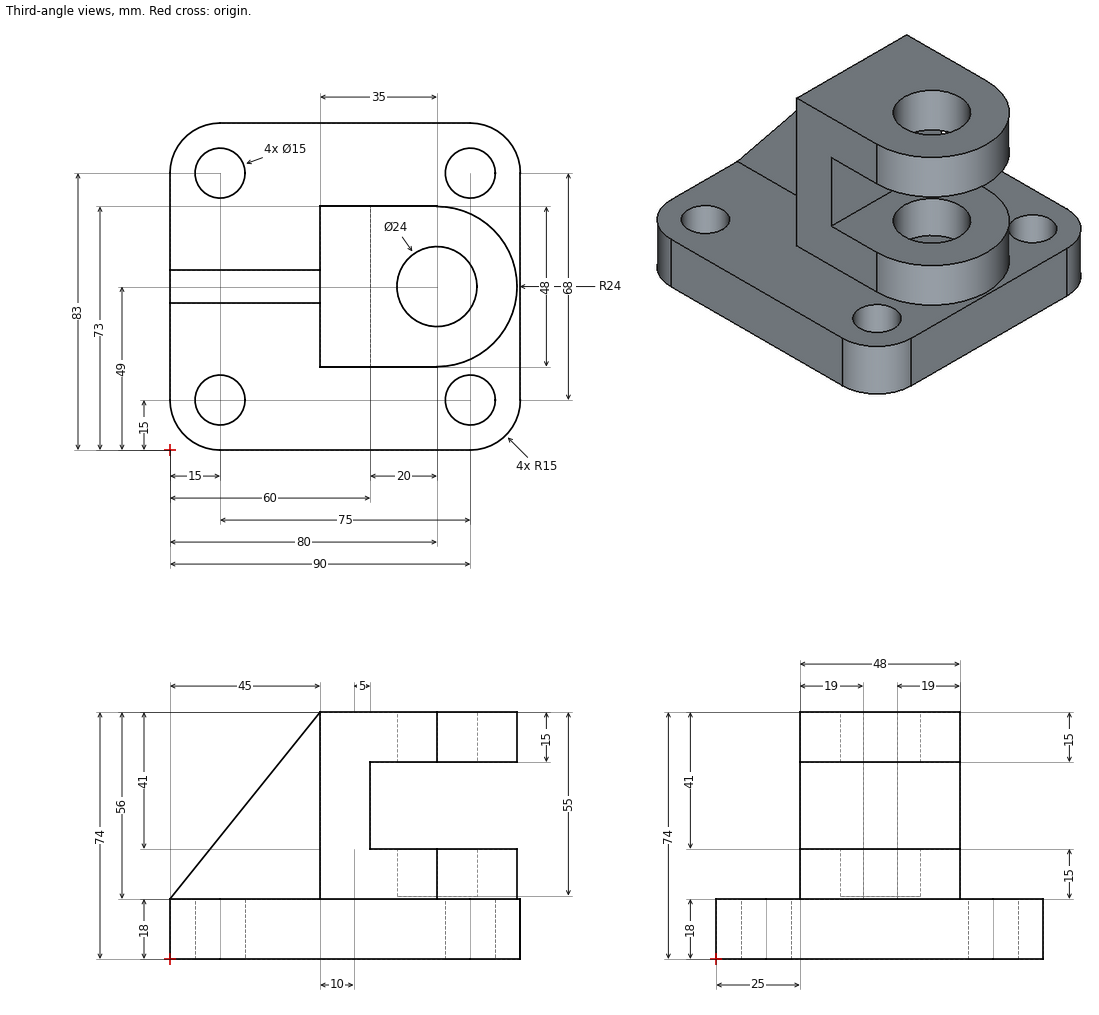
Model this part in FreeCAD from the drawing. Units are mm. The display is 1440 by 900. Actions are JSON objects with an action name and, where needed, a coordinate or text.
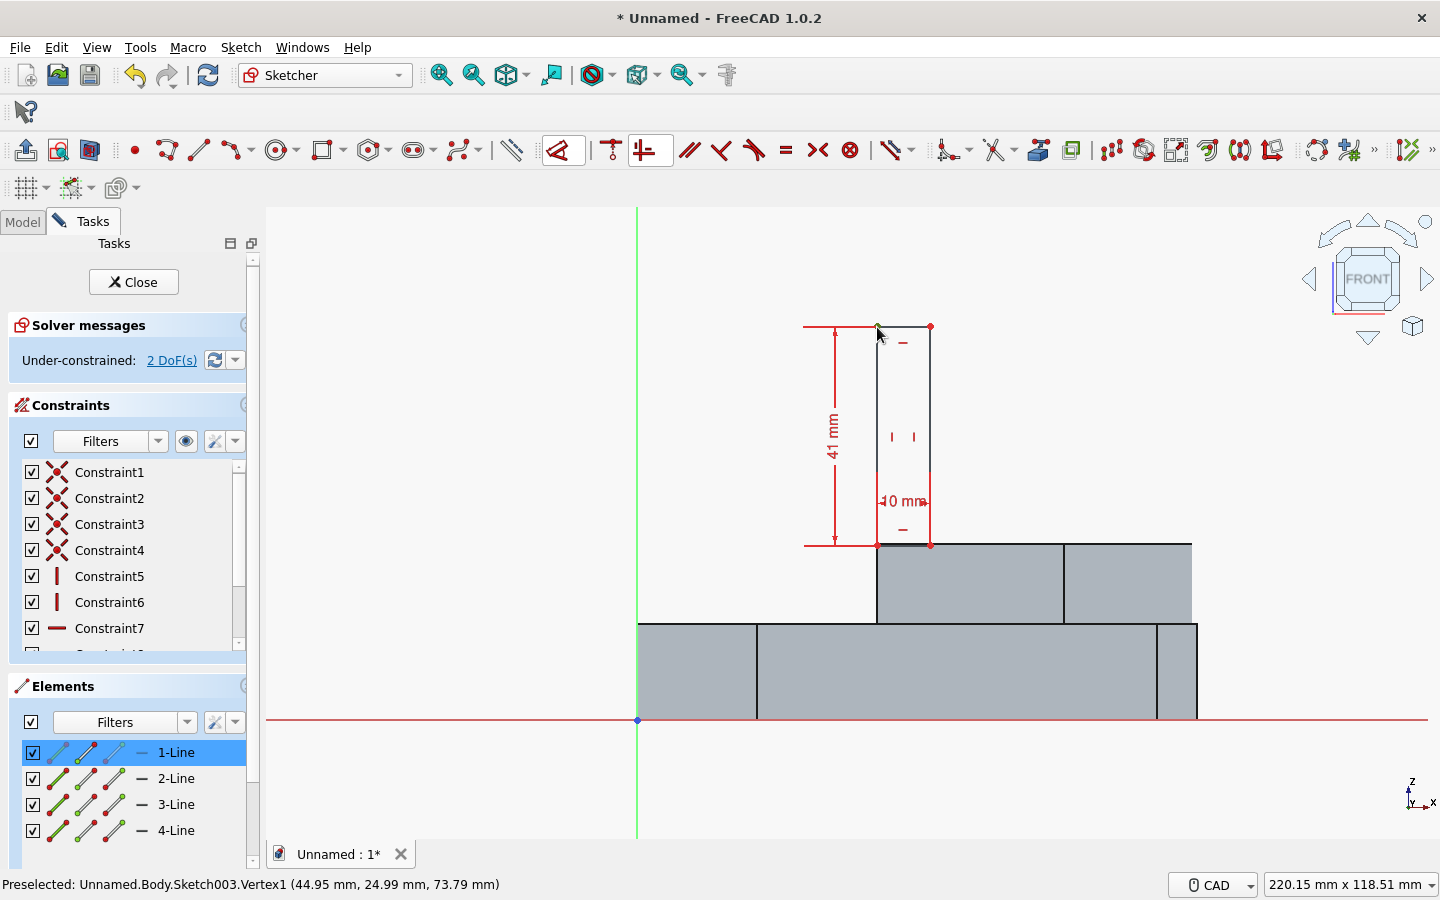
{"action": "left_click", "coordinate": [580, 150]}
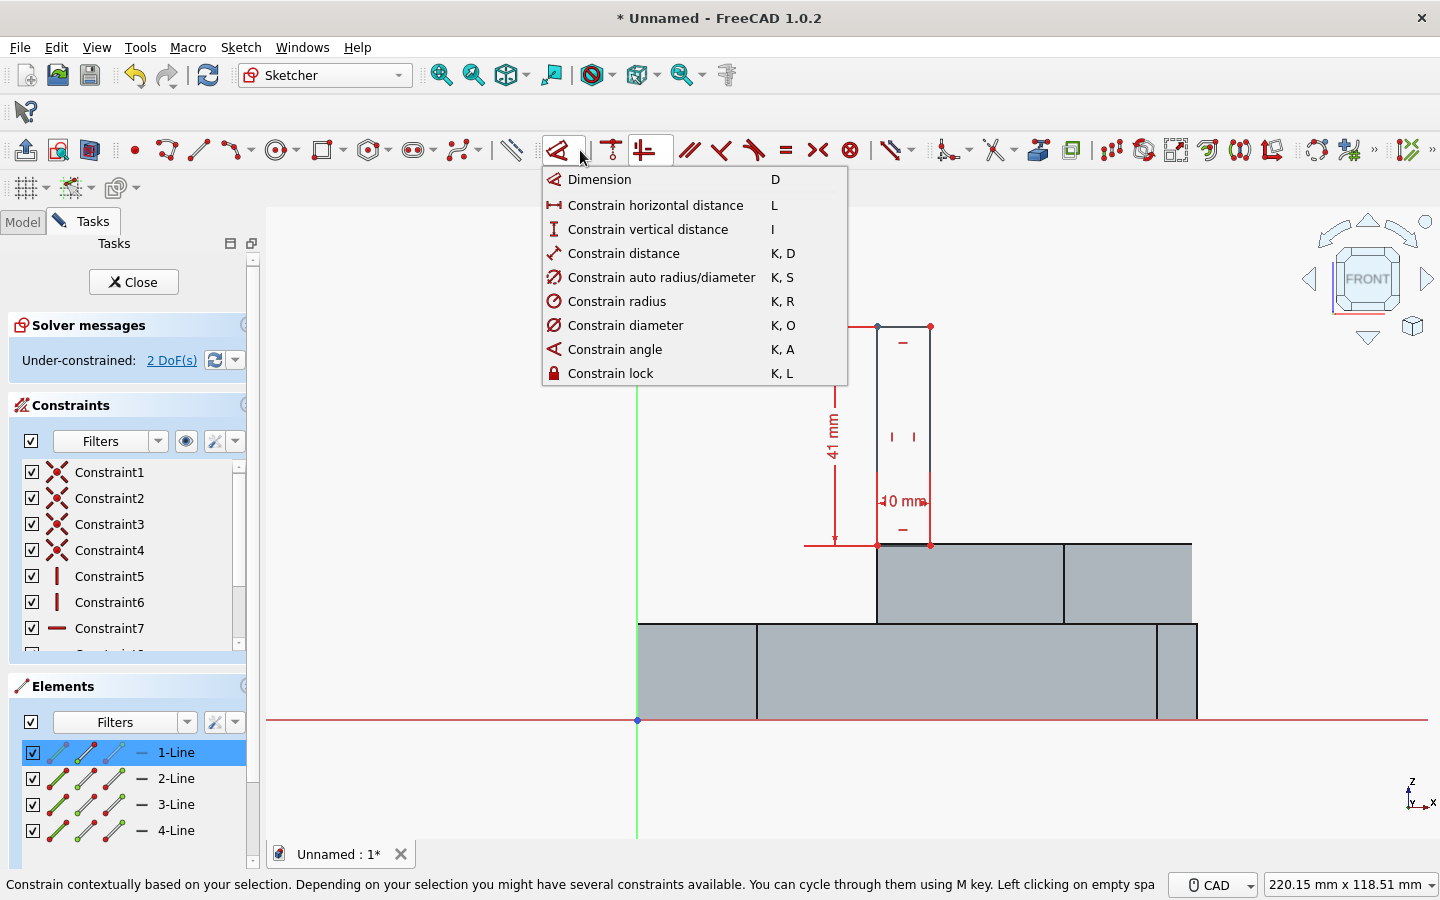
{"action": "left_click", "coordinate": [695, 205]}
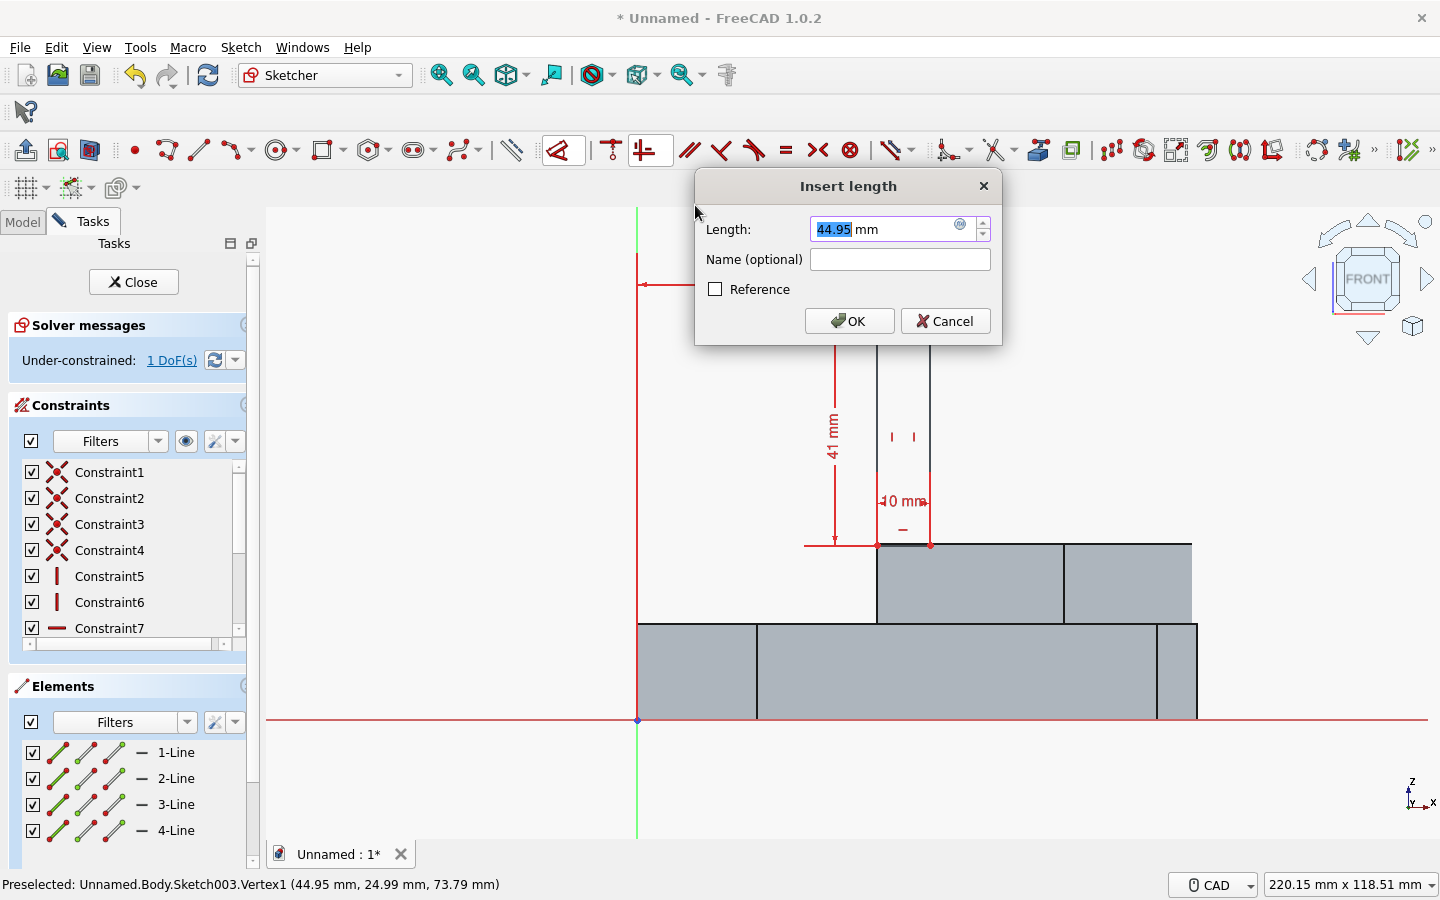
{"action": "type", "text": "45"}
{"action": "key", "text": "Return"}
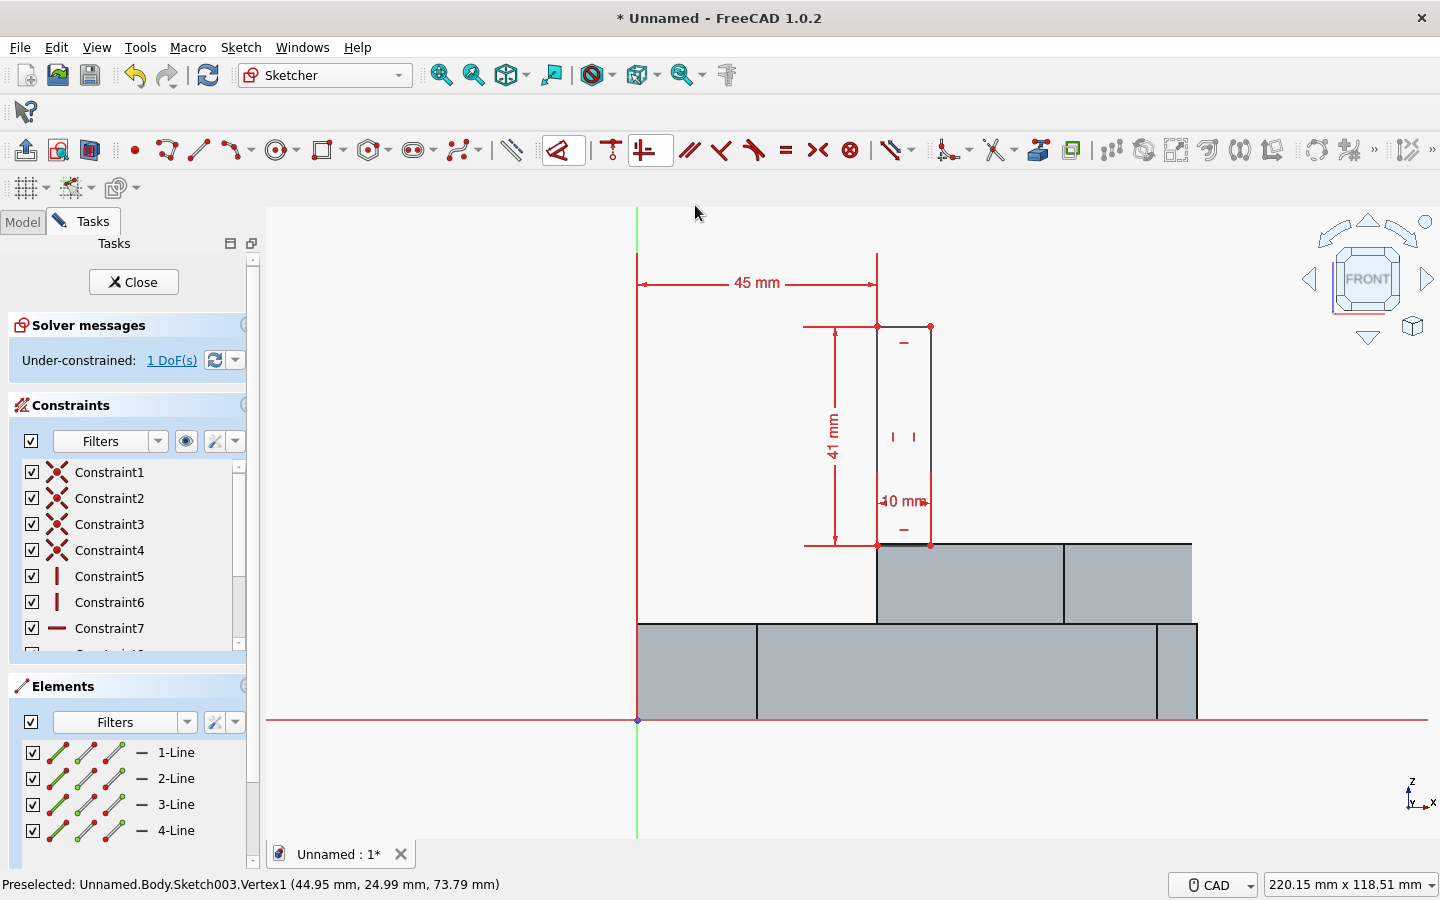
{"action": "left_click", "coordinate": [877, 327]}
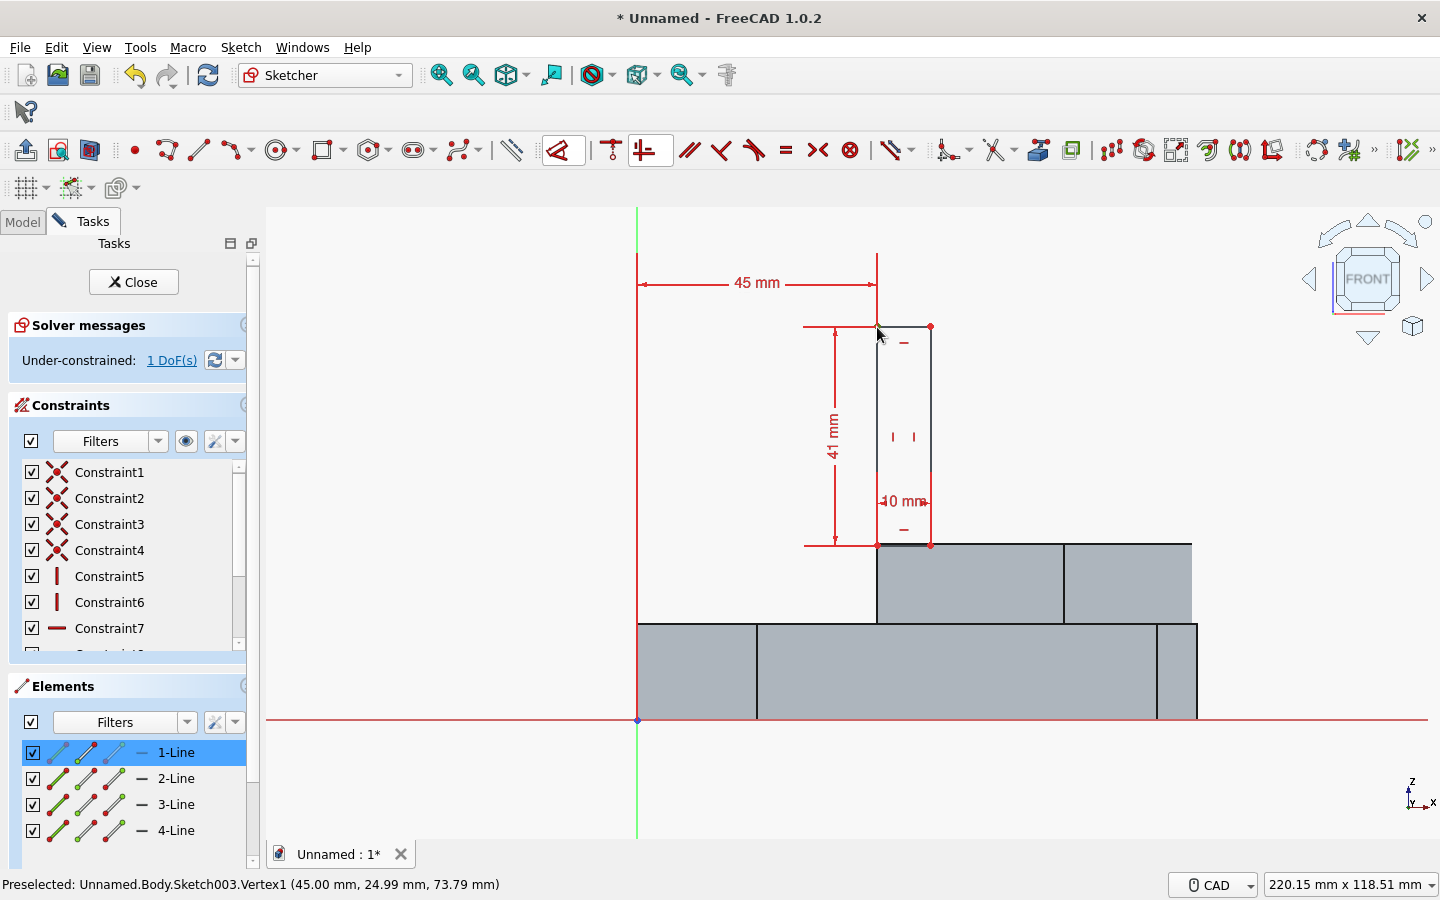
{"action": "key", "text": "i"}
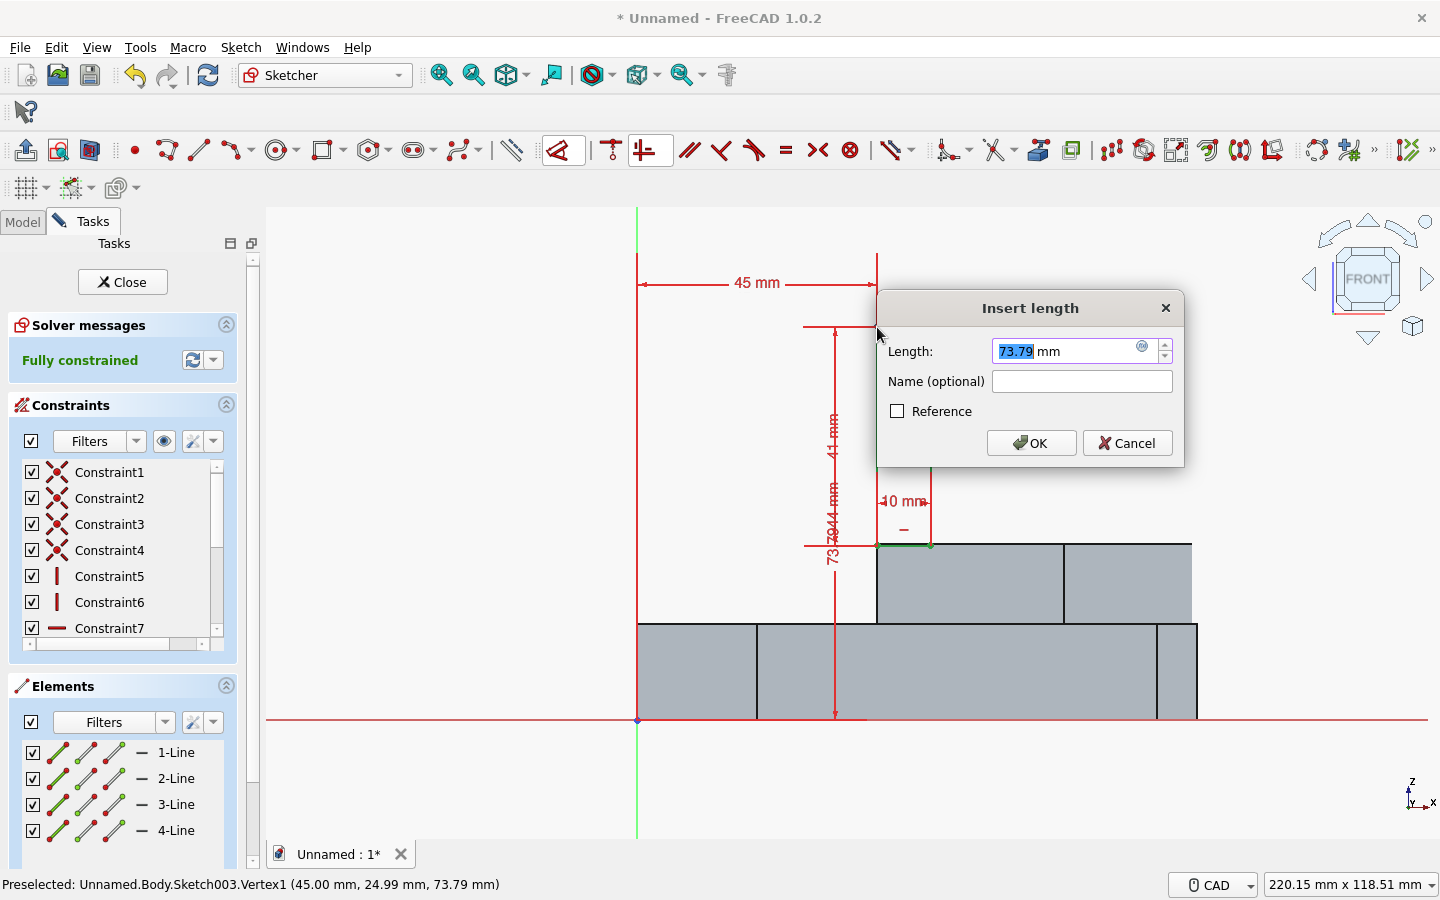
{"action": "type", "text": "74"}
{"action": "key", "text": "Return"}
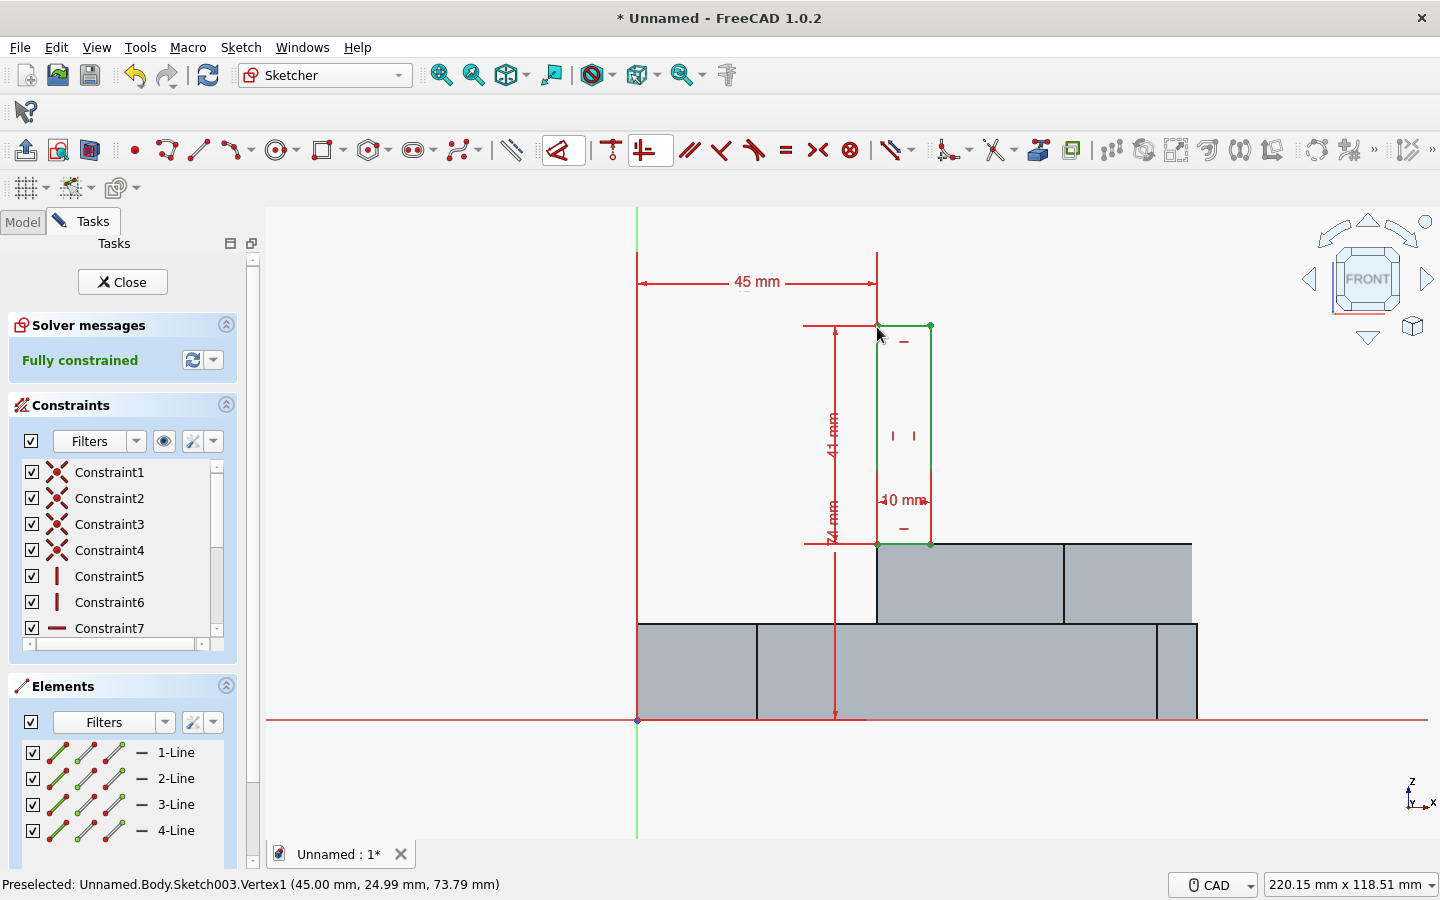
{"action": "left_click", "coordinate": [123, 282]}